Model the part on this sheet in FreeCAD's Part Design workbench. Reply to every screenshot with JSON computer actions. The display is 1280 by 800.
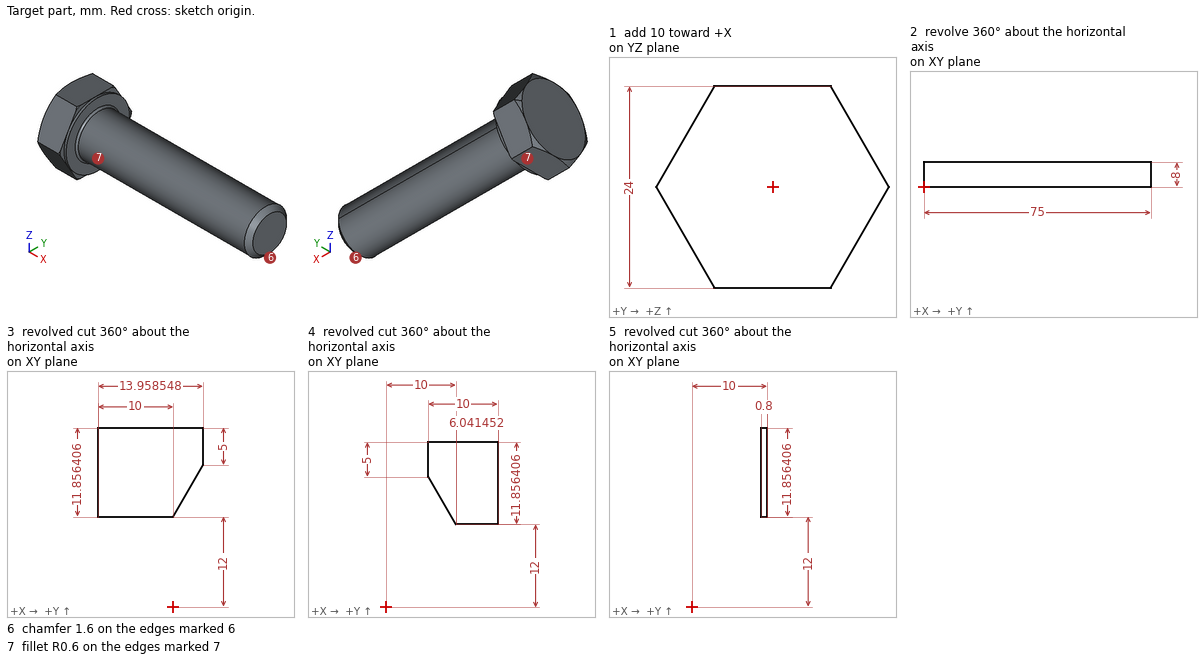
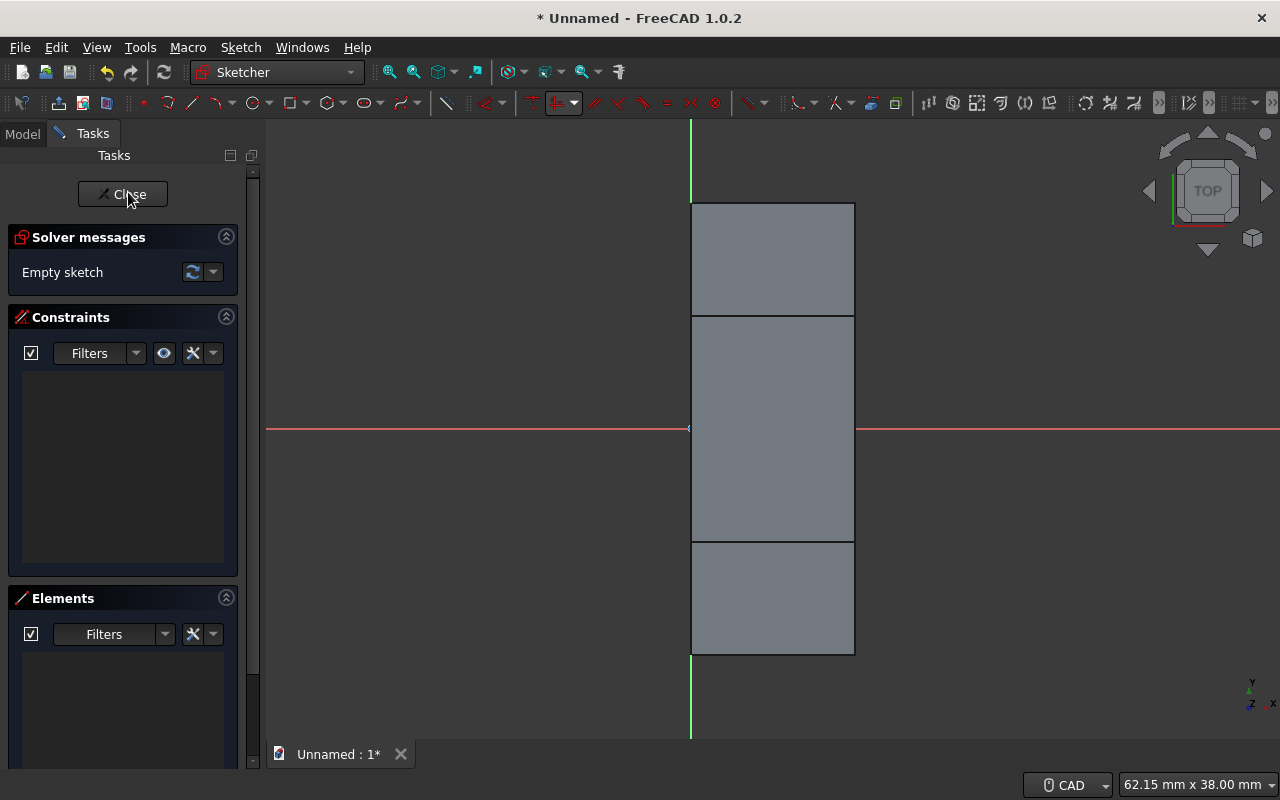
{"action": "left_click", "coordinate": [108, 104]}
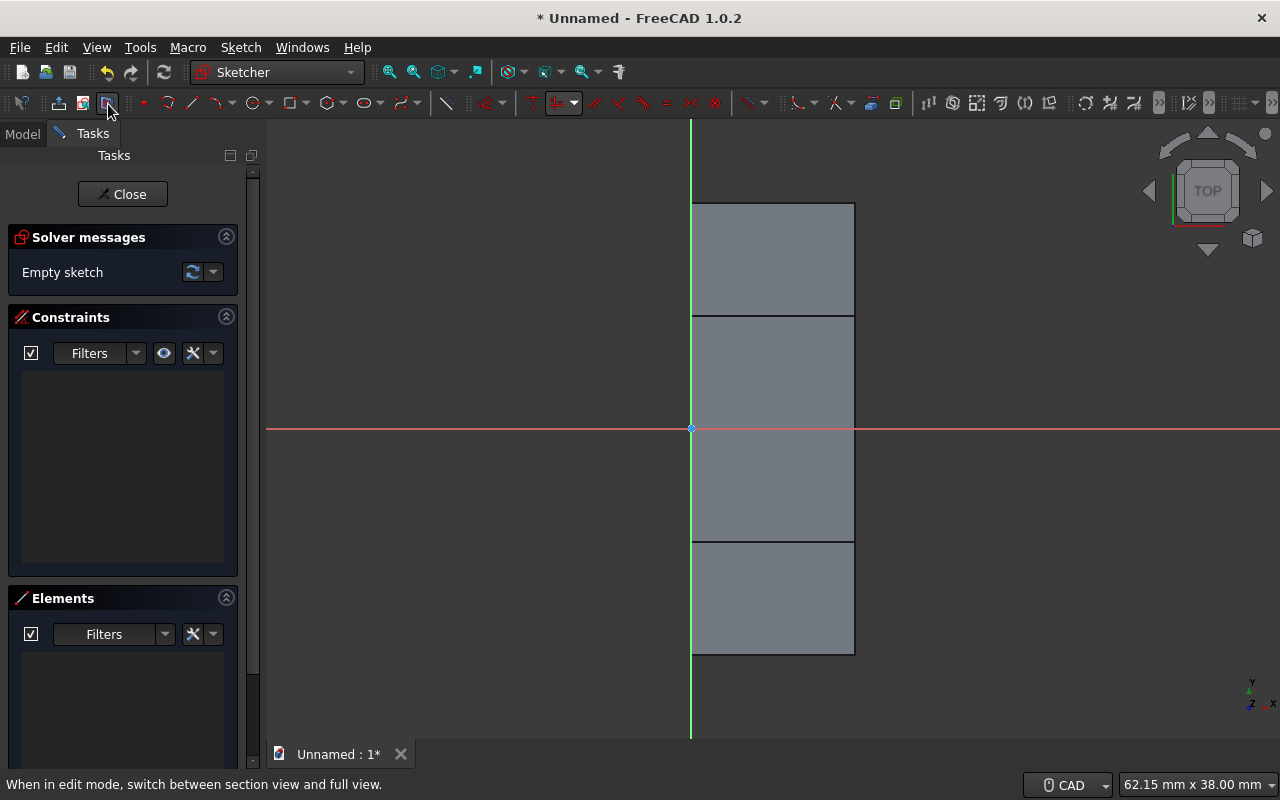
{"action": "scroll", "coordinate": [294, 482], "scroll_direction": "down", "scroll_amount": 4}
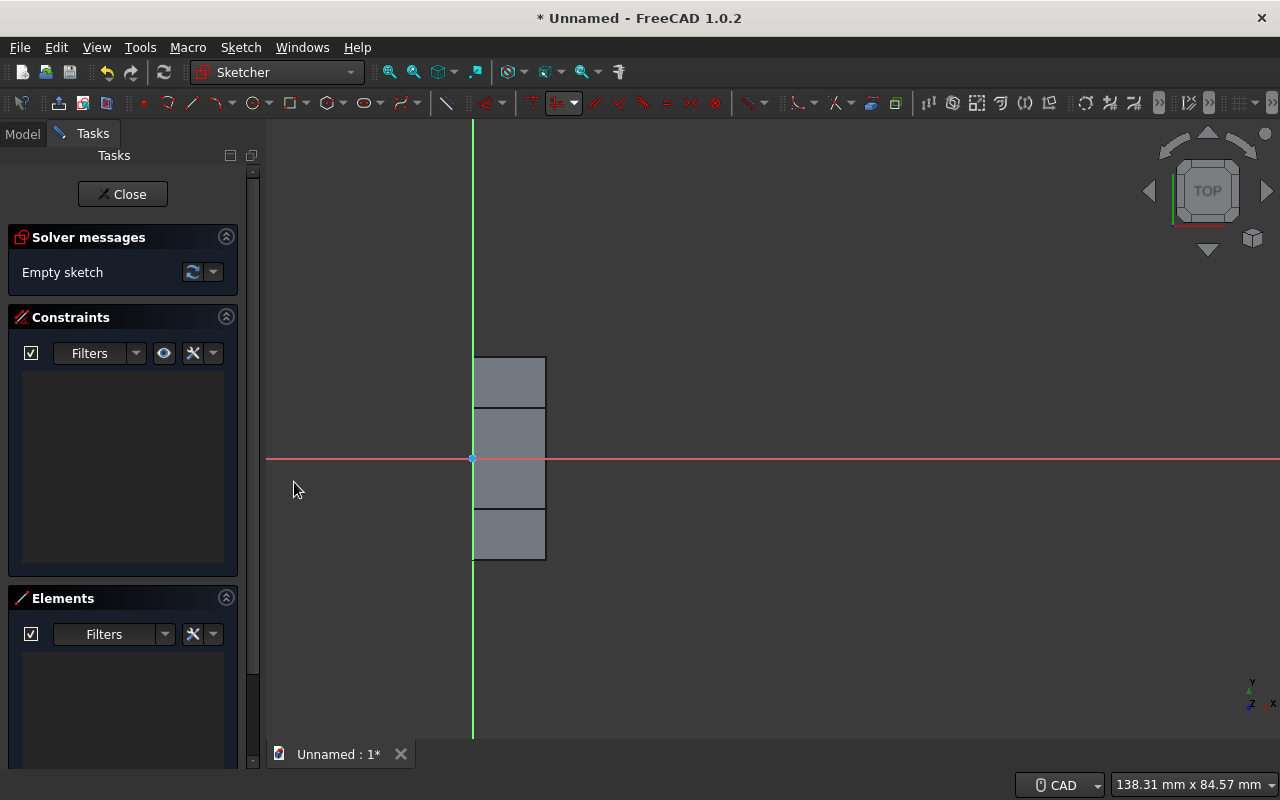
{"action": "left_click", "coordinate": [290, 104]}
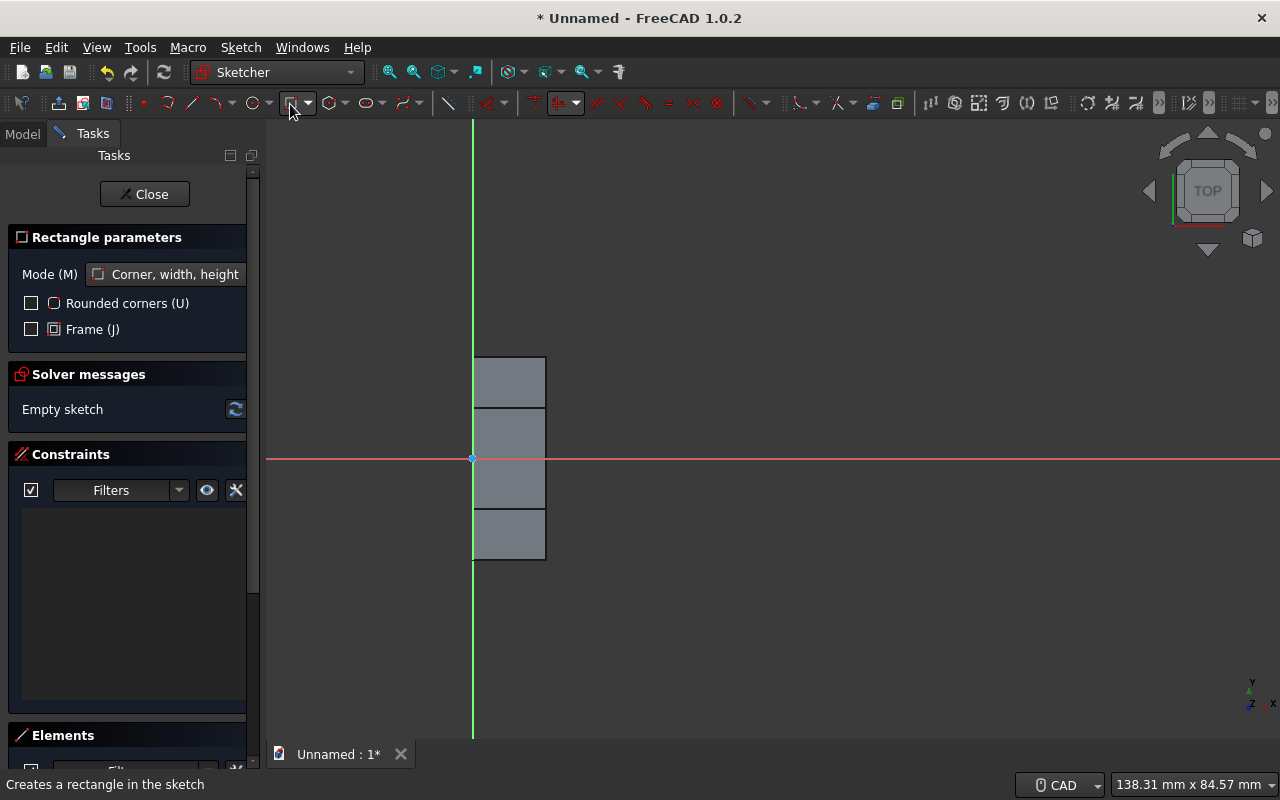
{"action": "left_click", "coordinate": [473, 459]}
{"action": "mouse_move", "coordinate": [1022, 400]}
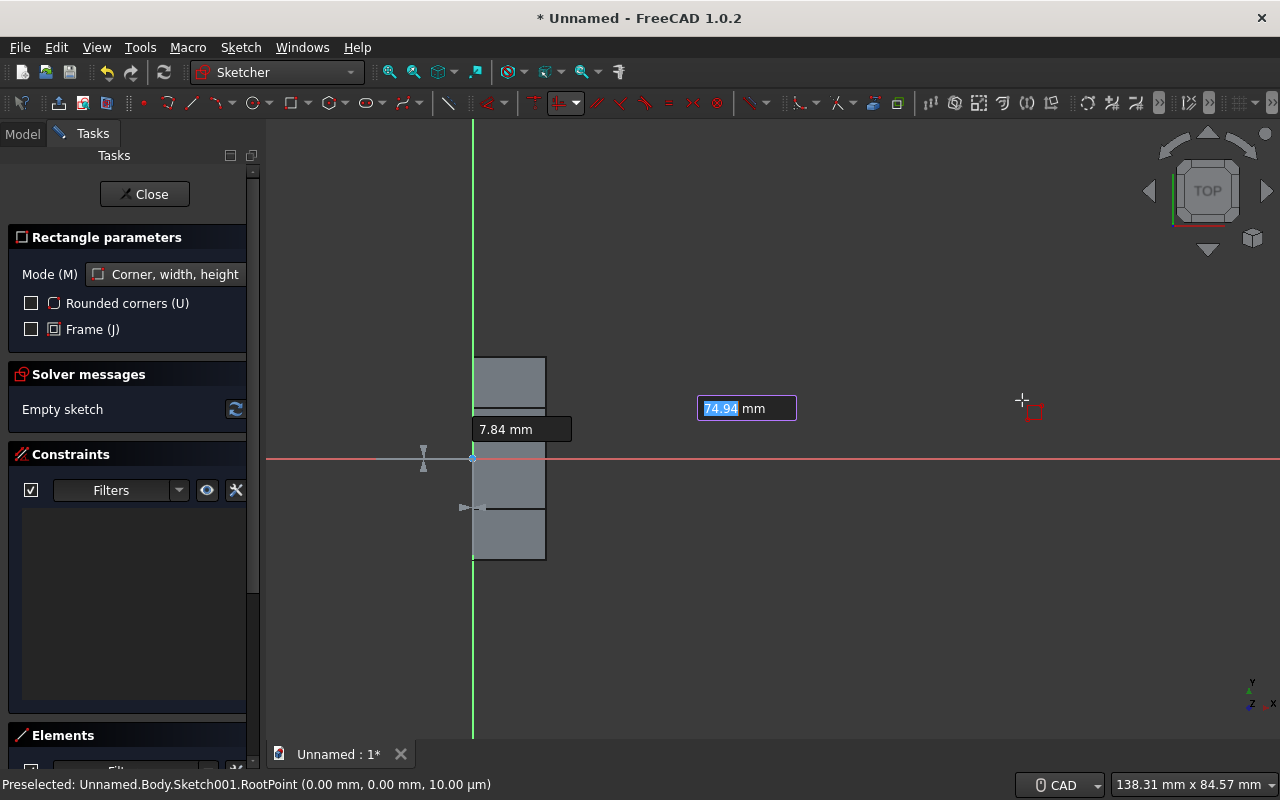
{"action": "type", "text": "75"}
{"action": "key", "text": "Tab"}
{"action": "type", "text": "8"}
{"action": "key", "text": "Return"}
{"action": "key", "text": "Escape"}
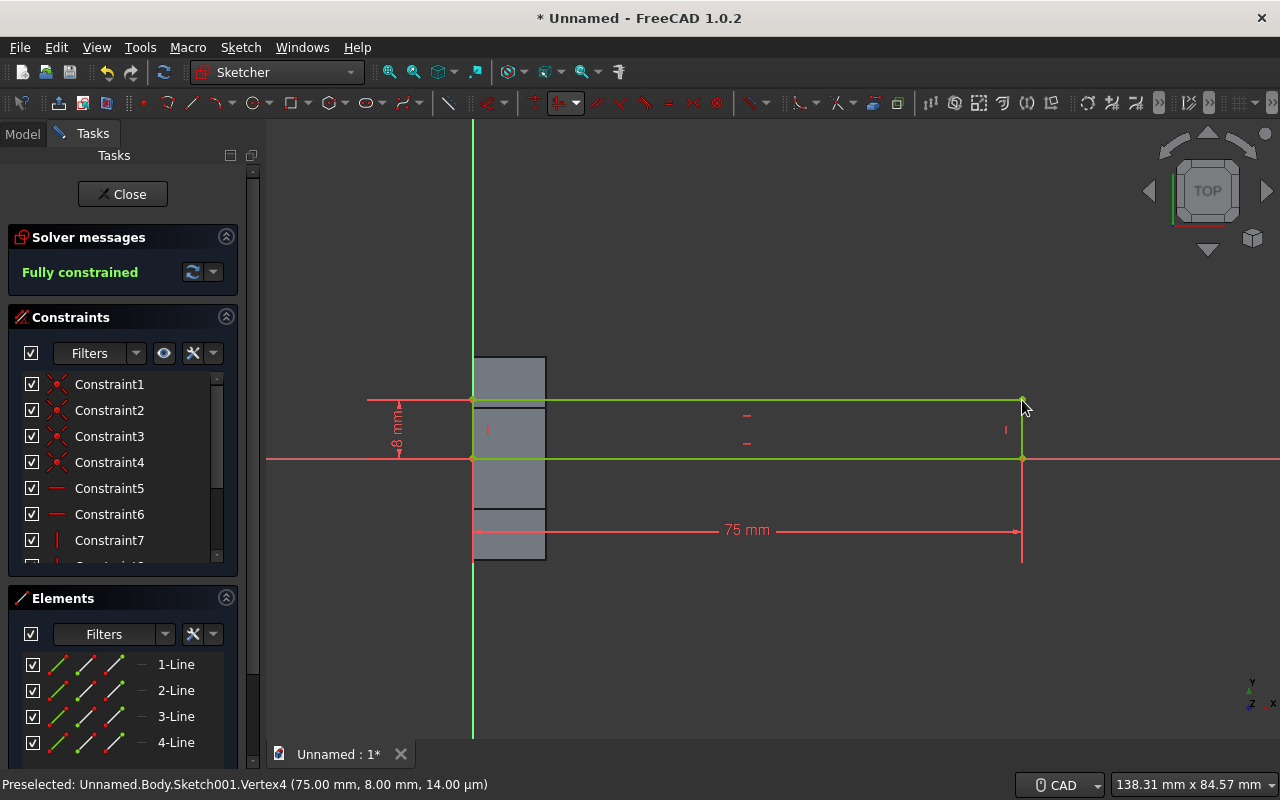
{"action": "left_click", "coordinate": [123, 194]}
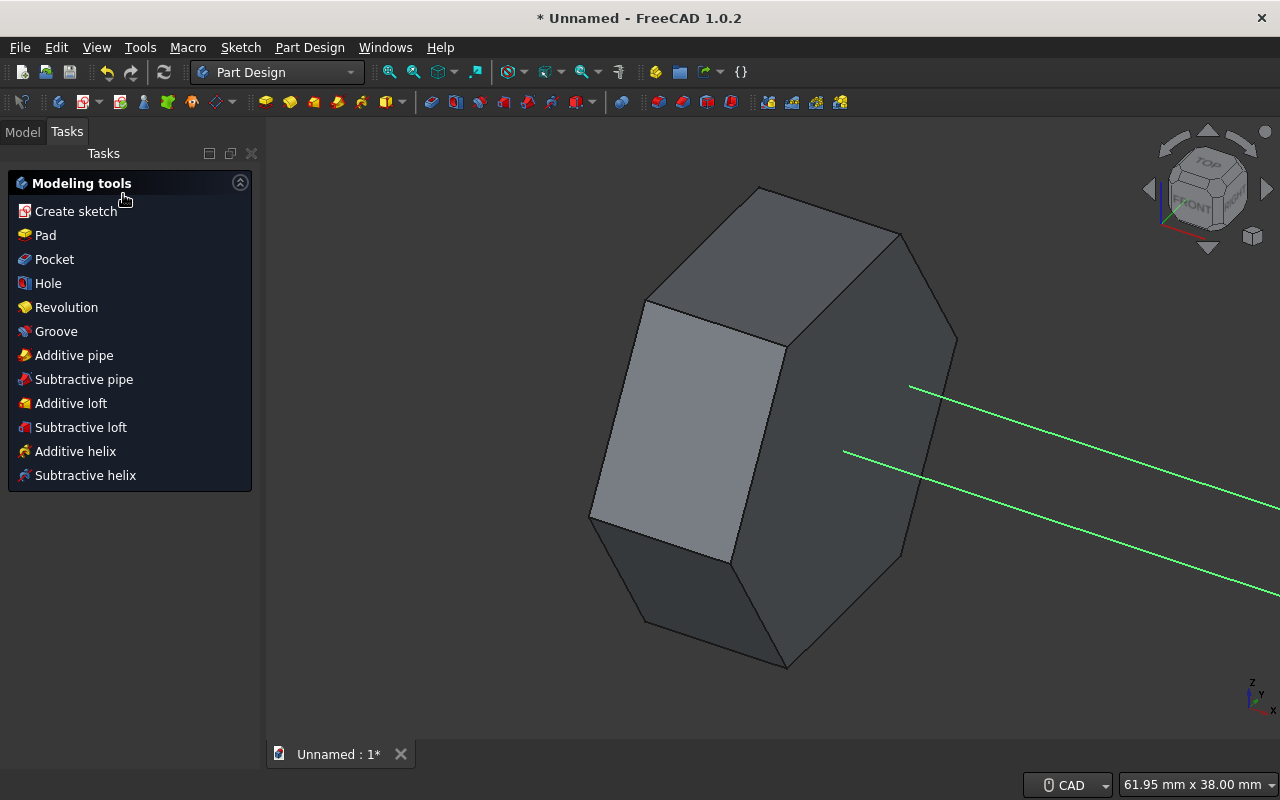
{"action": "left_click", "coordinate": [290, 102]}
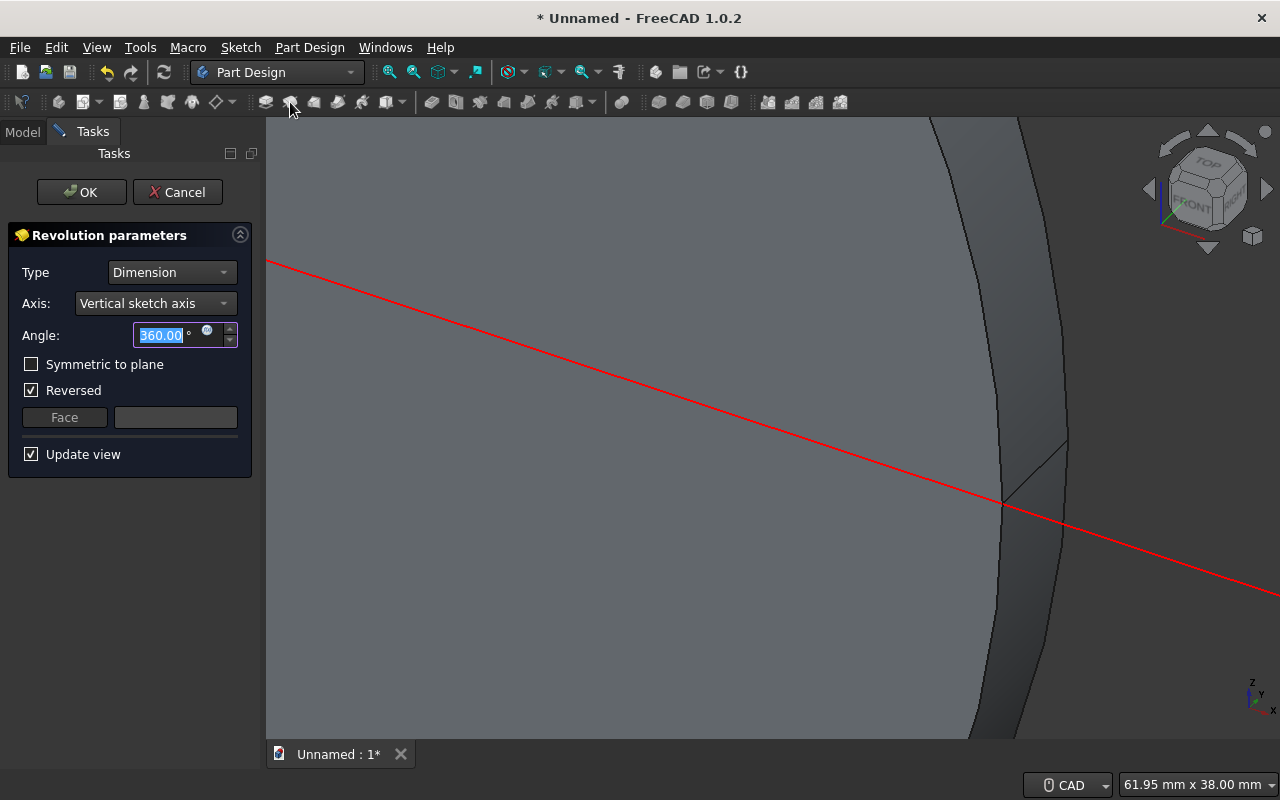
{"action": "left_click", "coordinate": [156, 304]}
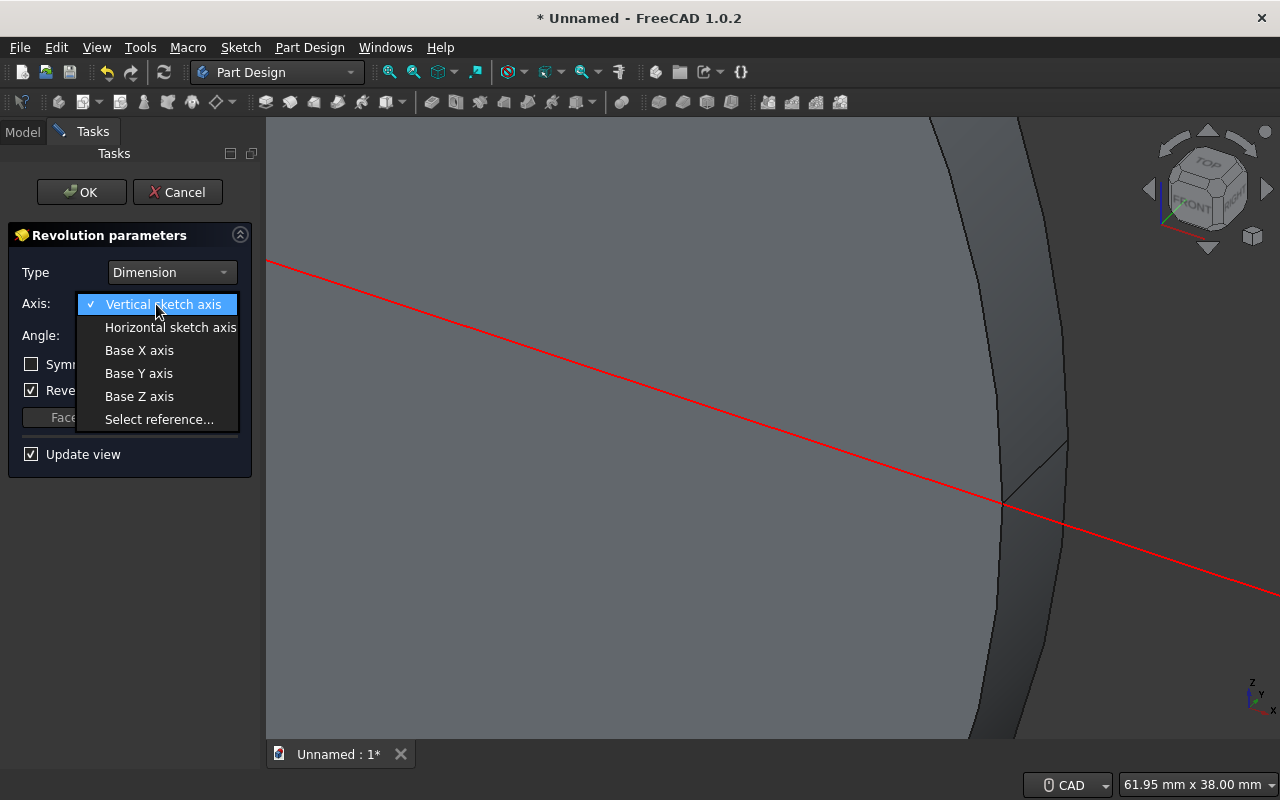
{"action": "left_click", "coordinate": [156, 328]}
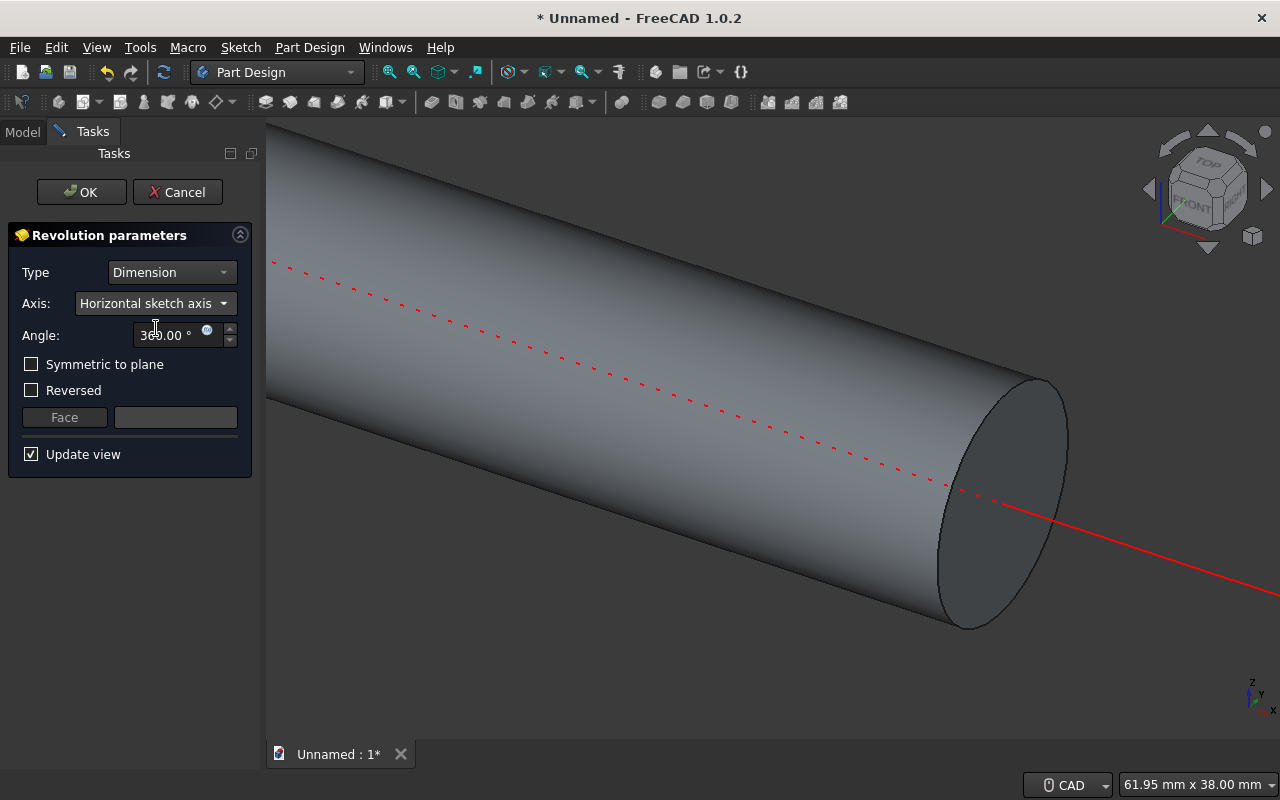
{"action": "left_click", "coordinate": [82, 192]}